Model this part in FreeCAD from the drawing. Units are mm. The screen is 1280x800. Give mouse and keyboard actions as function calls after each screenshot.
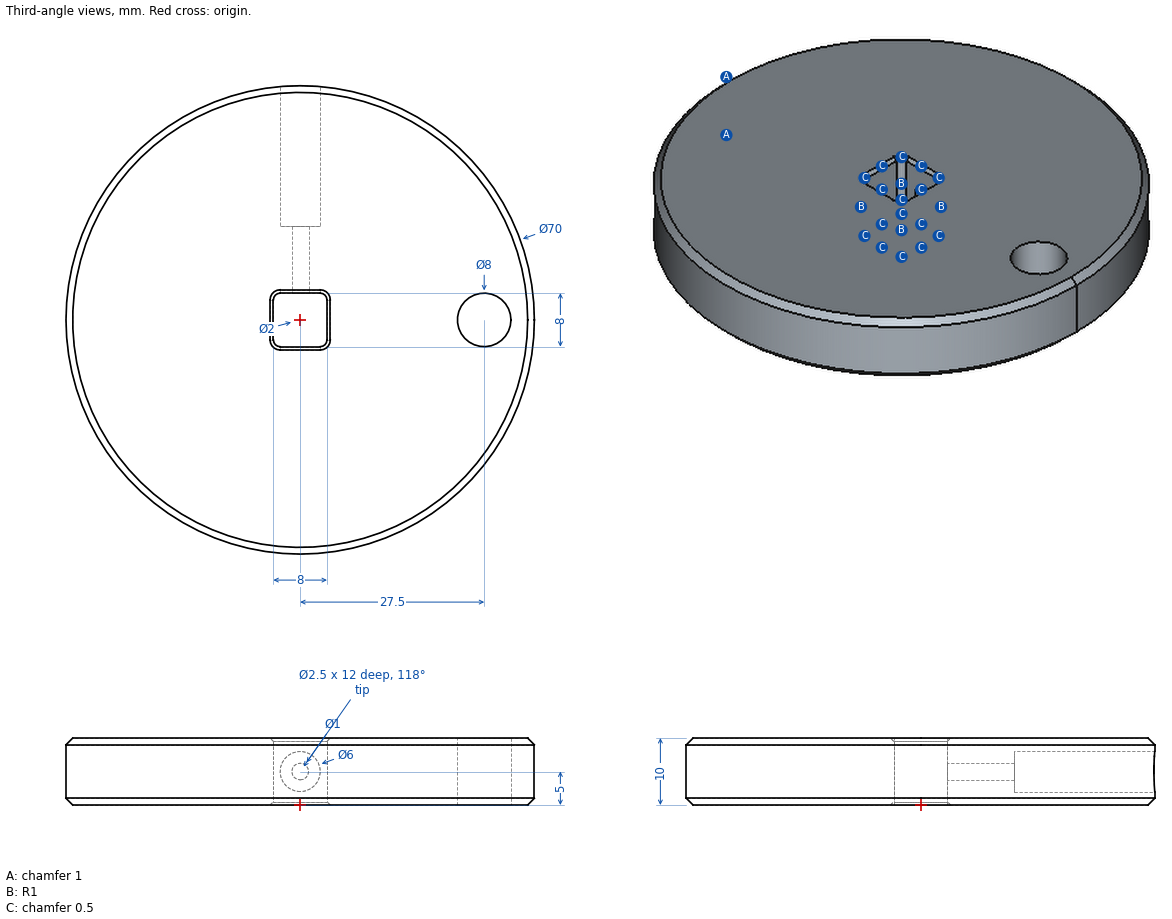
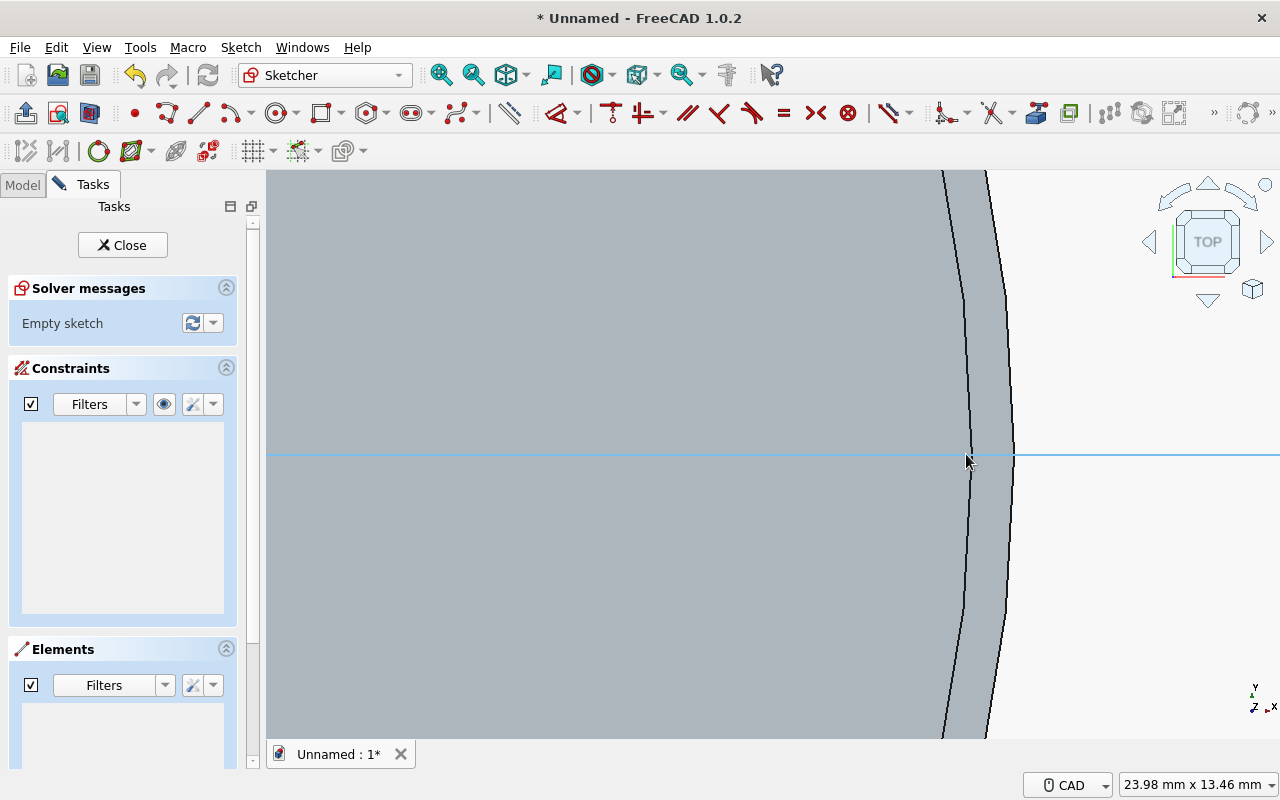
click(276, 114)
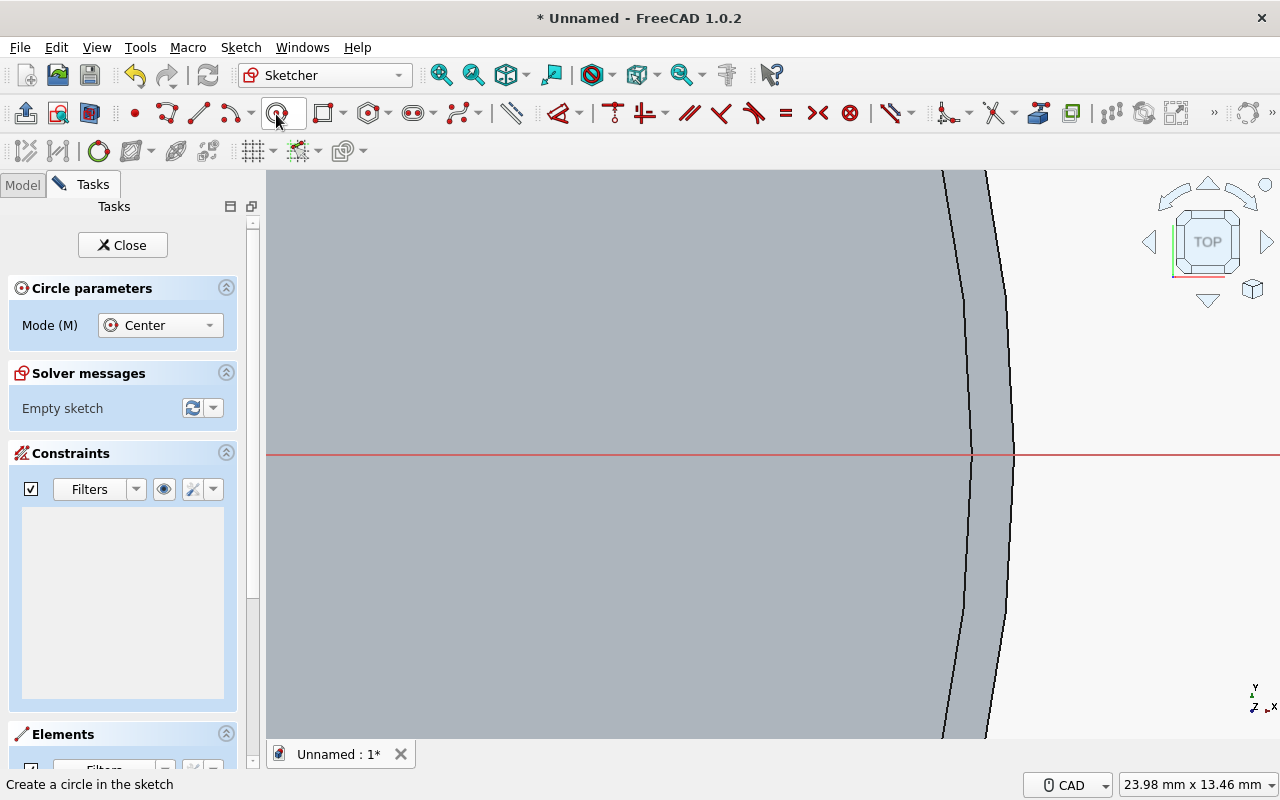
click(697, 454)
click(817, 335)
key(Escape)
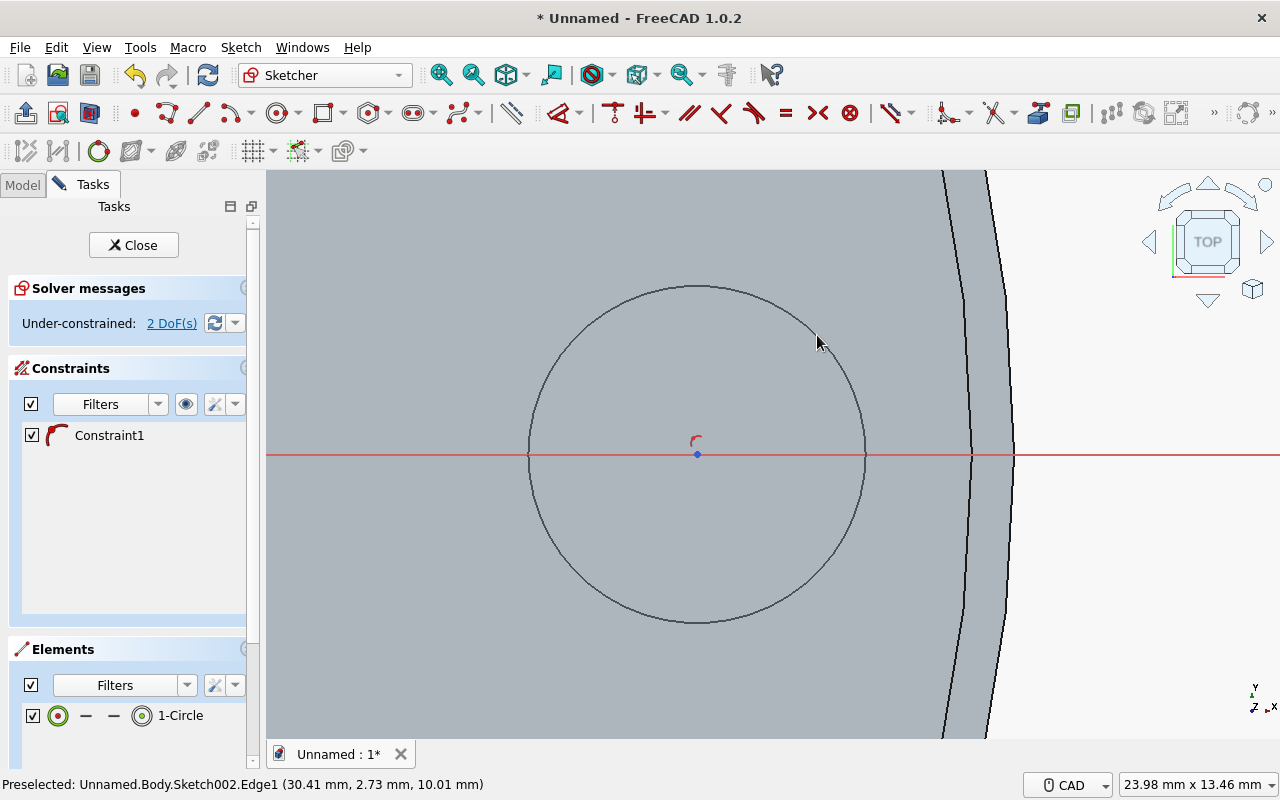
click(558, 114)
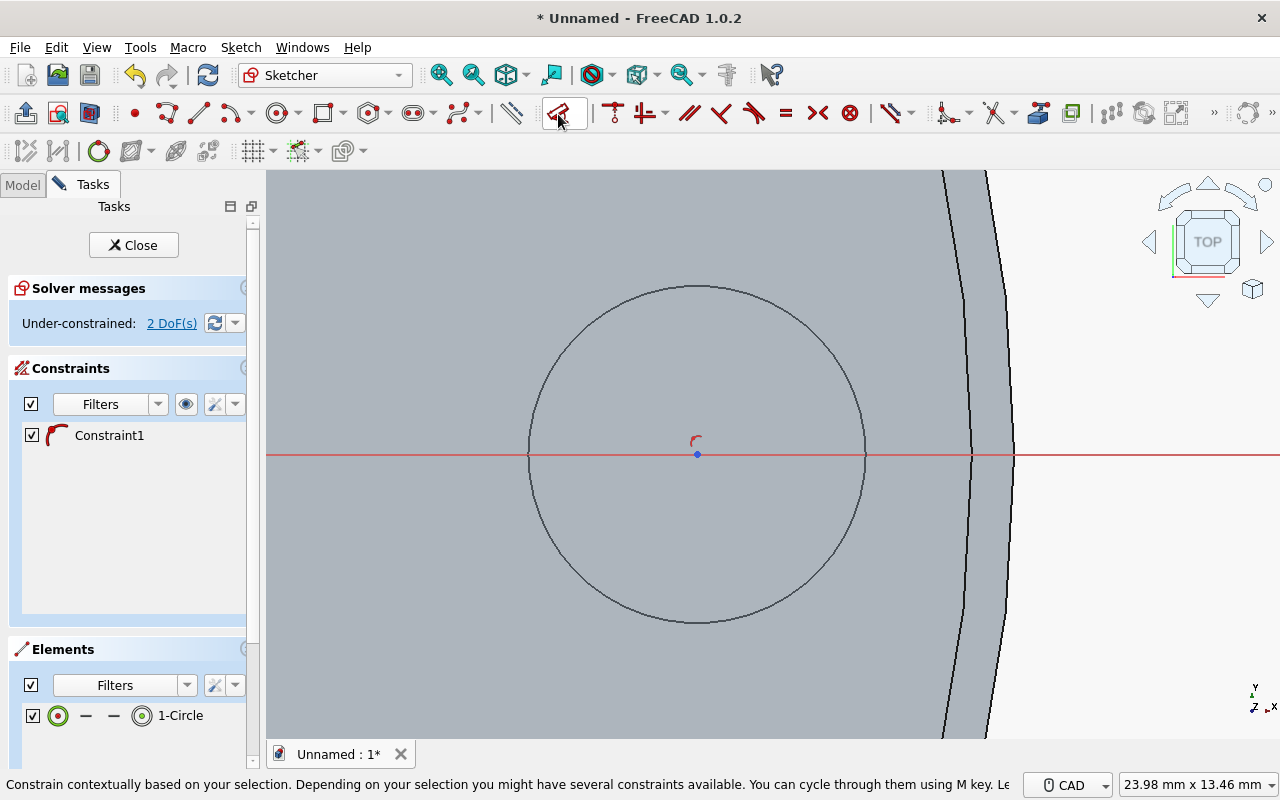
click(816, 335)
click(839, 312)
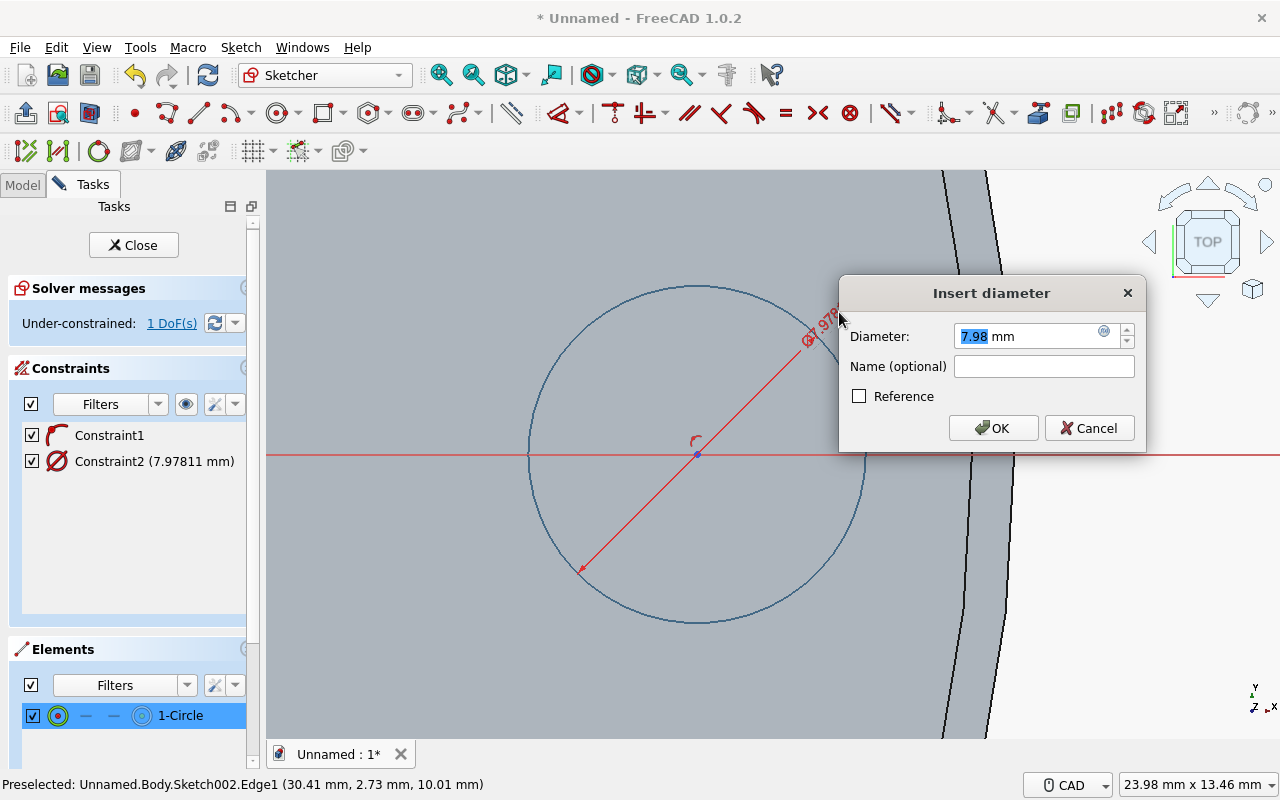
text(8)
key(Return)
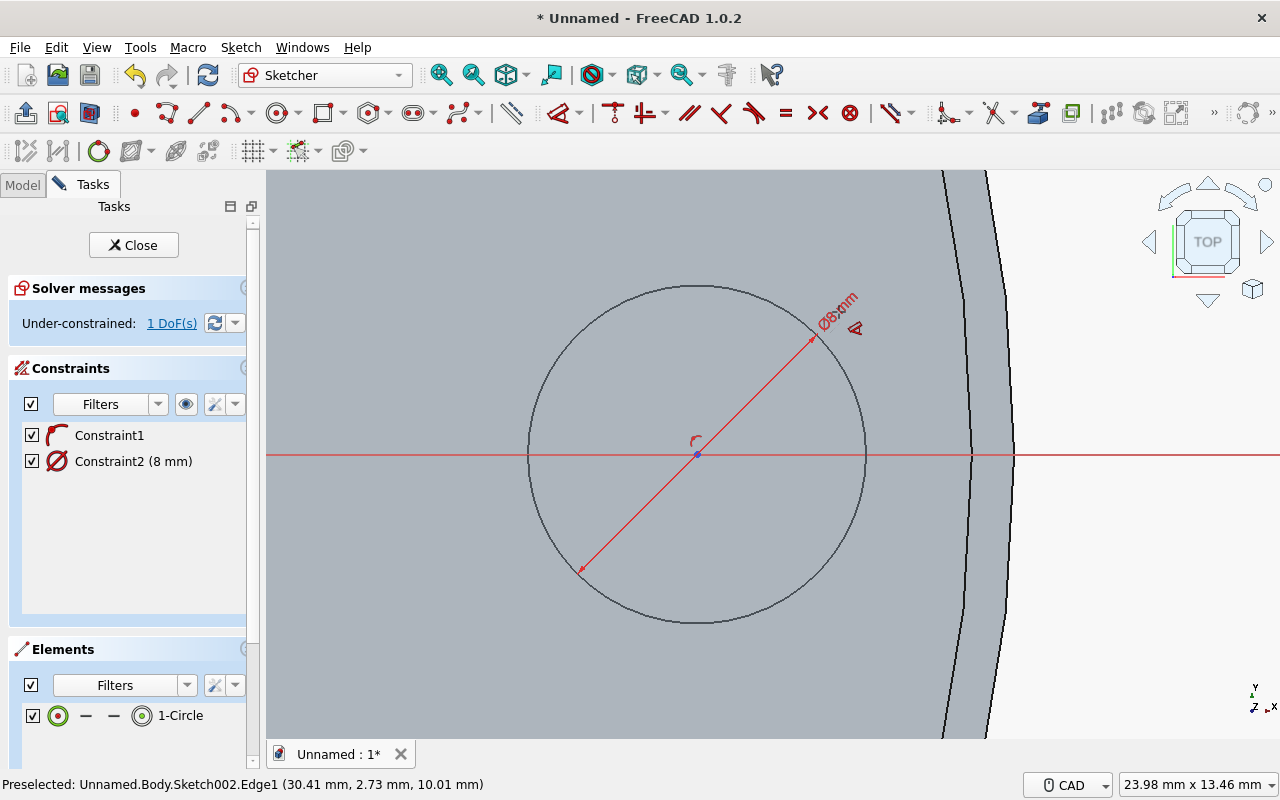
click(697, 454)
click(495, 488)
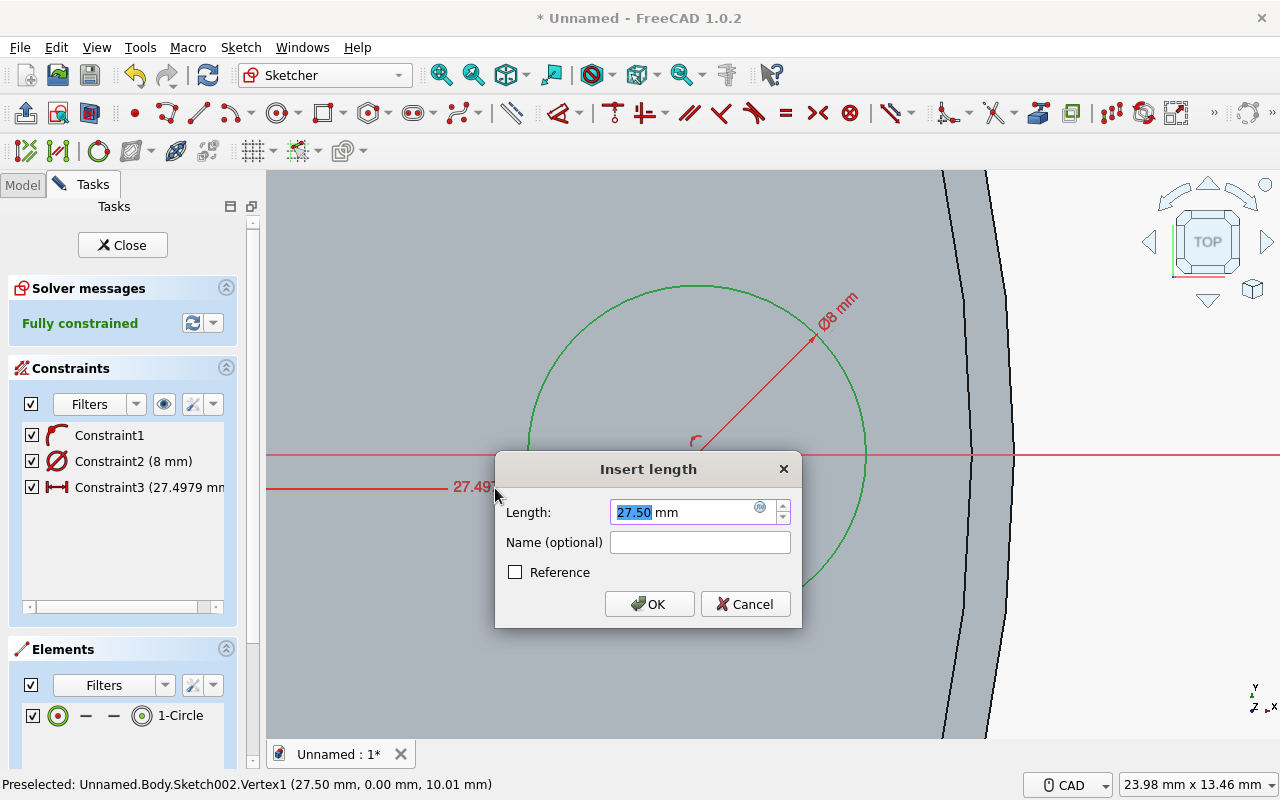
text(27.5)
key(Return)
key(Escape)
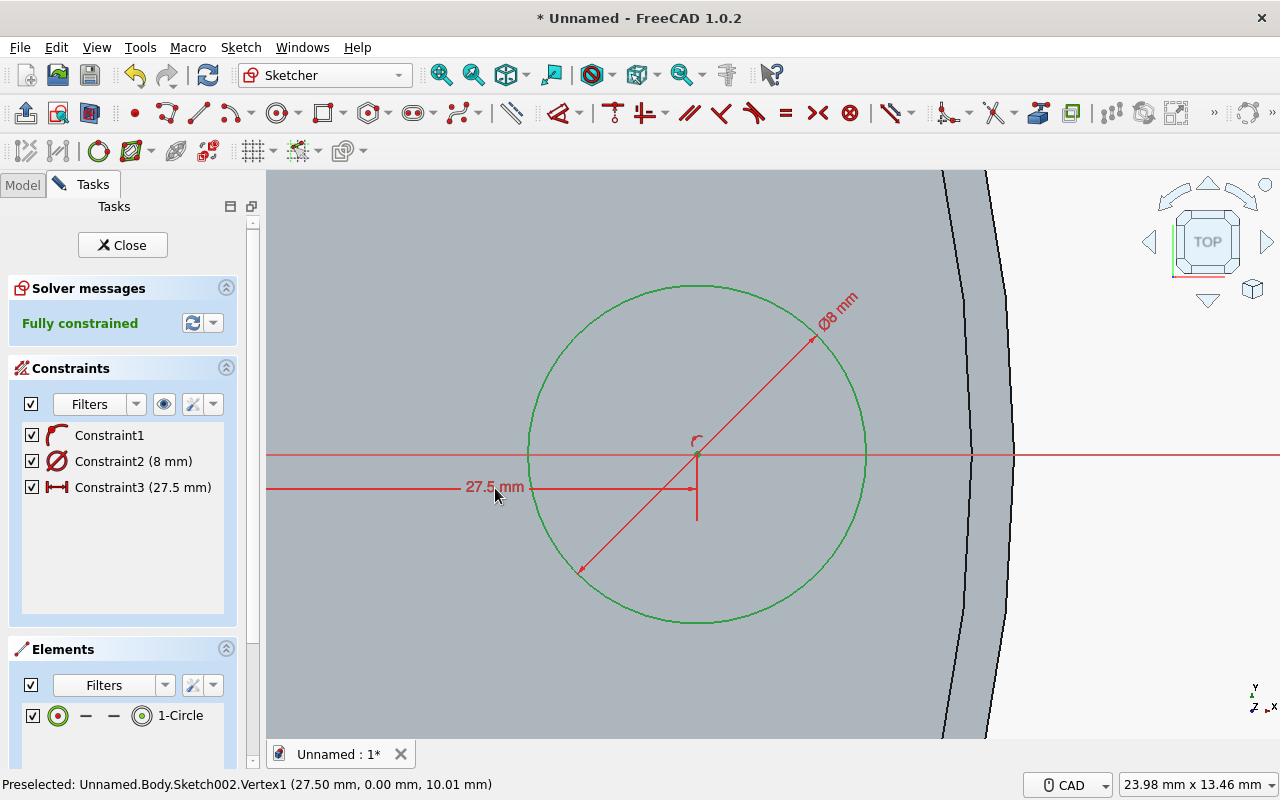
click(123, 245)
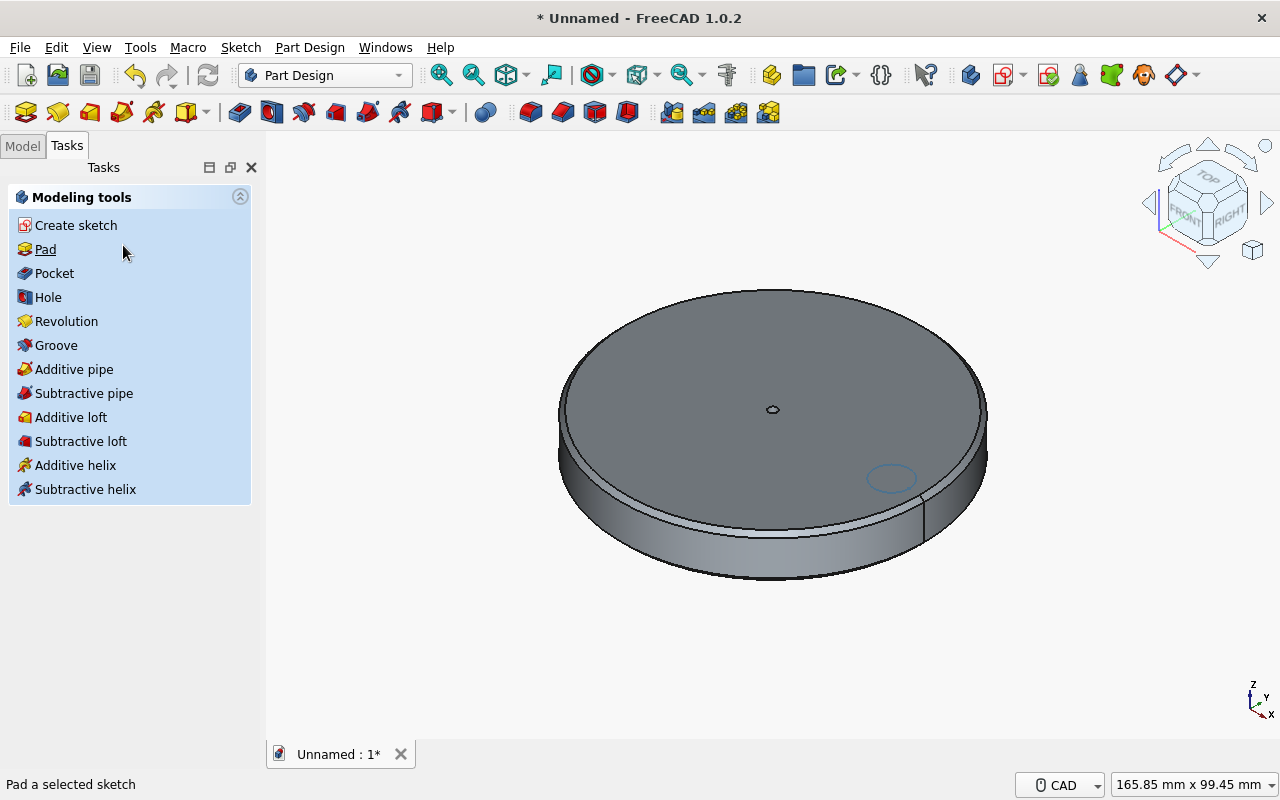
click(240, 112)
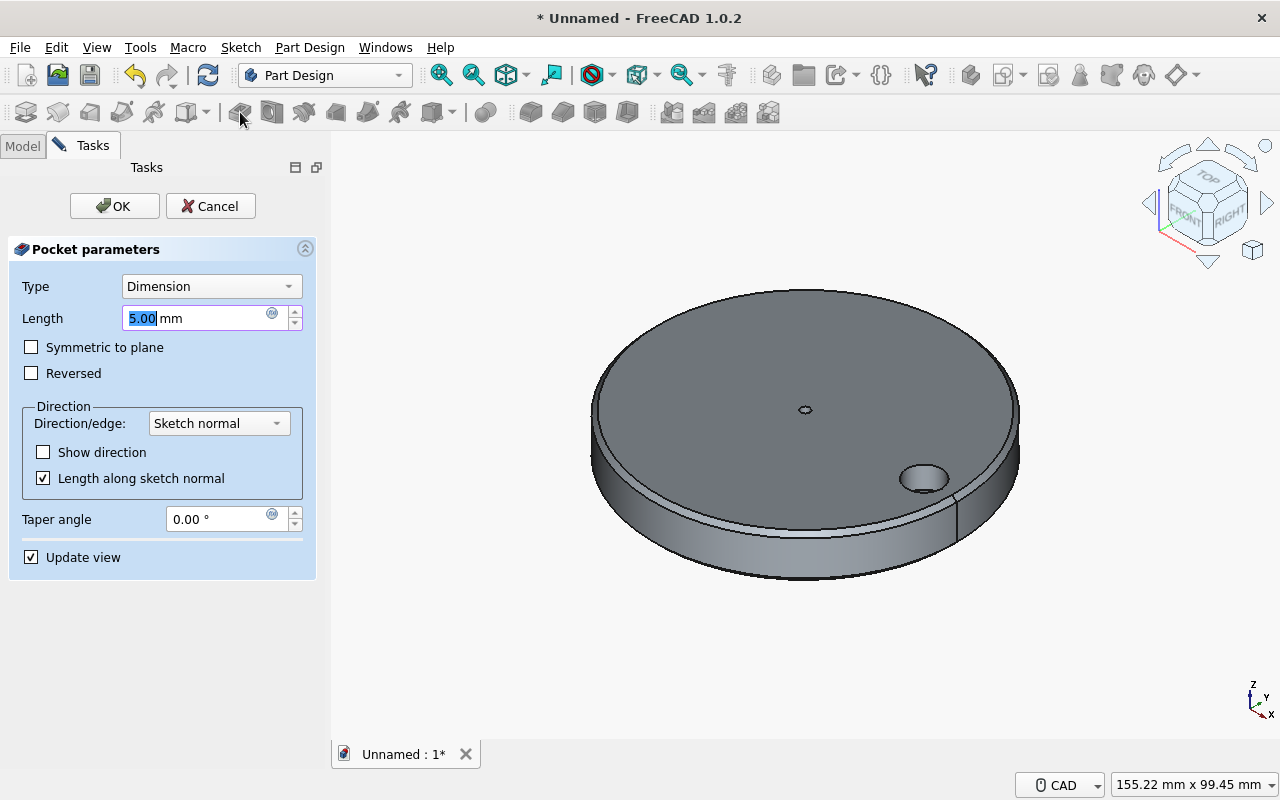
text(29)
key(Tab)